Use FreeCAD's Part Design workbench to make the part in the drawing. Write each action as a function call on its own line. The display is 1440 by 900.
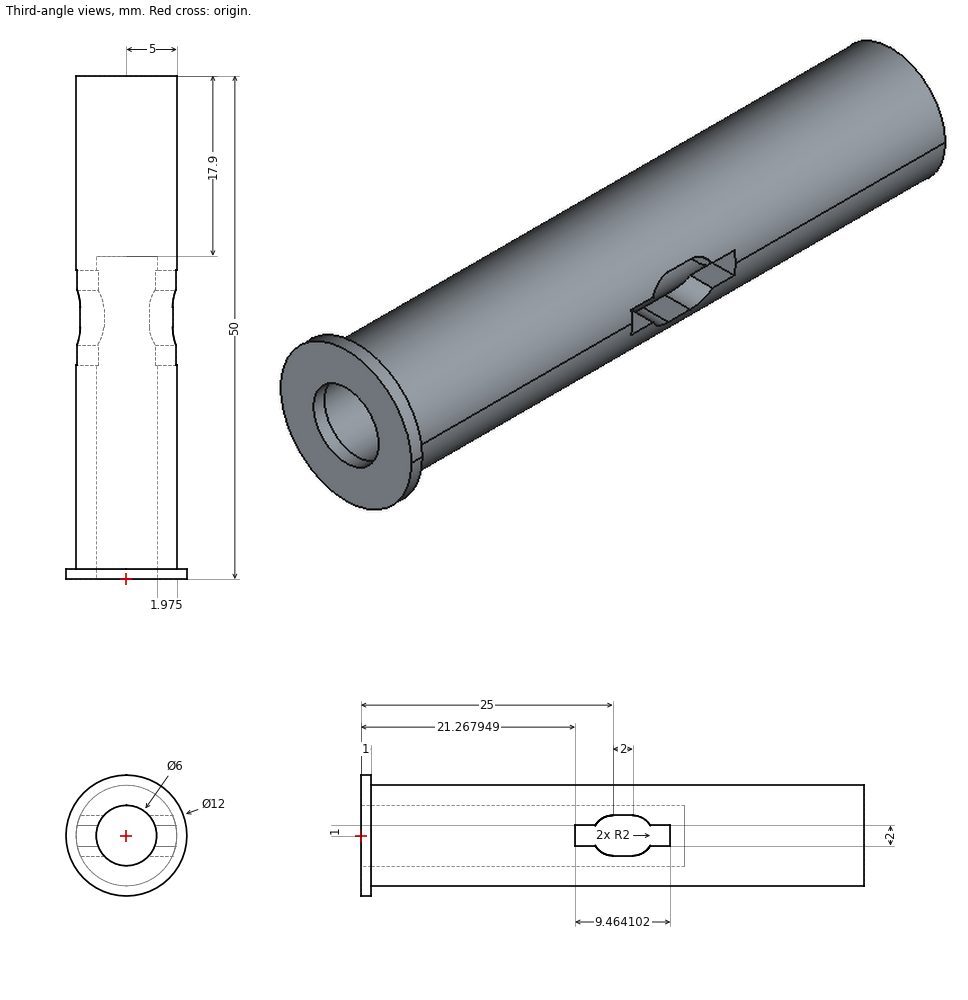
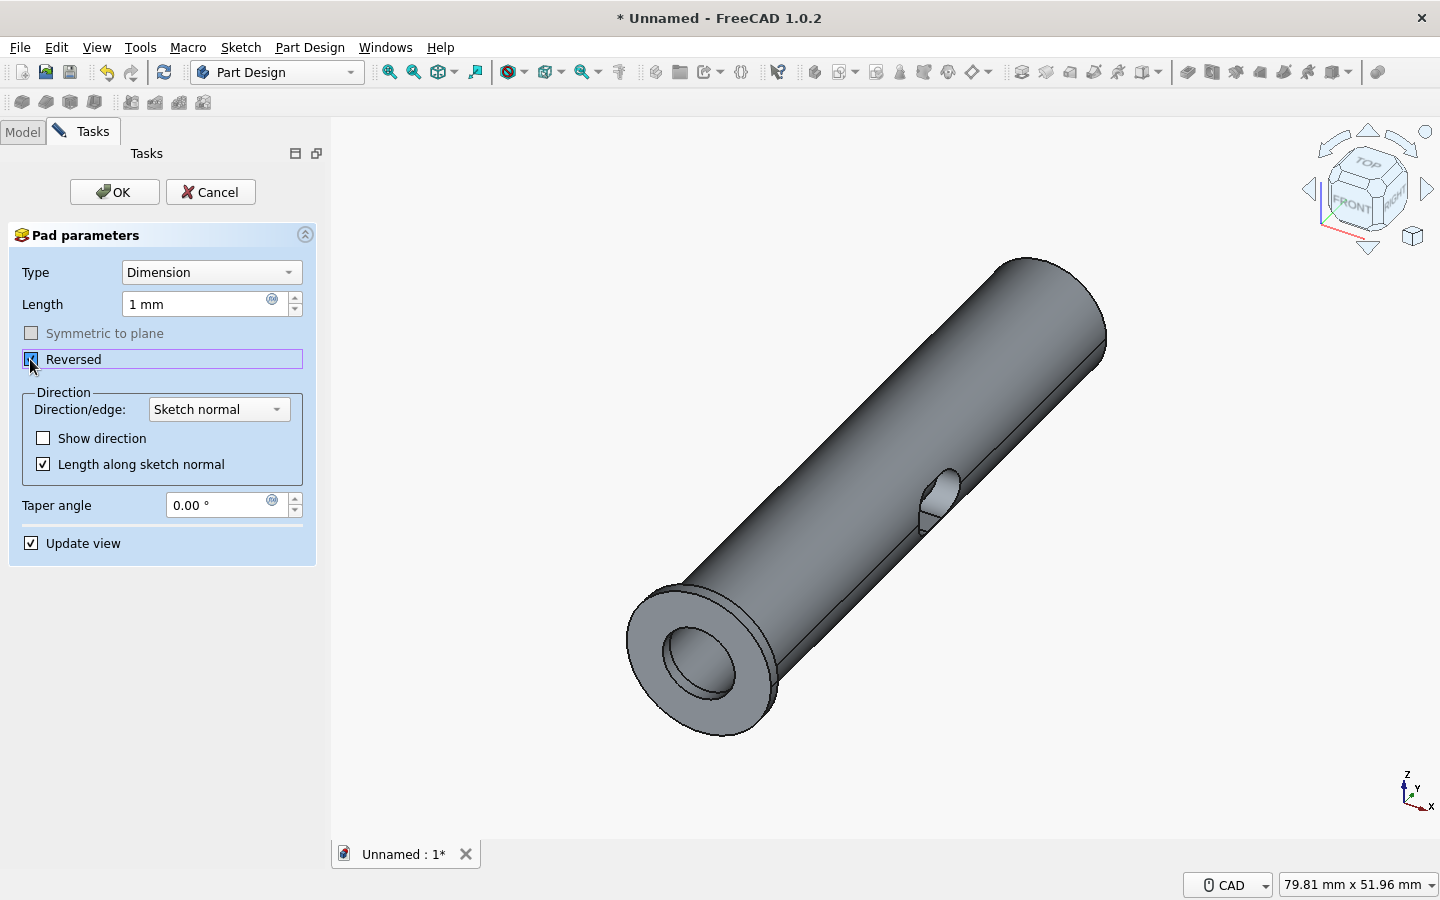
click(115, 192)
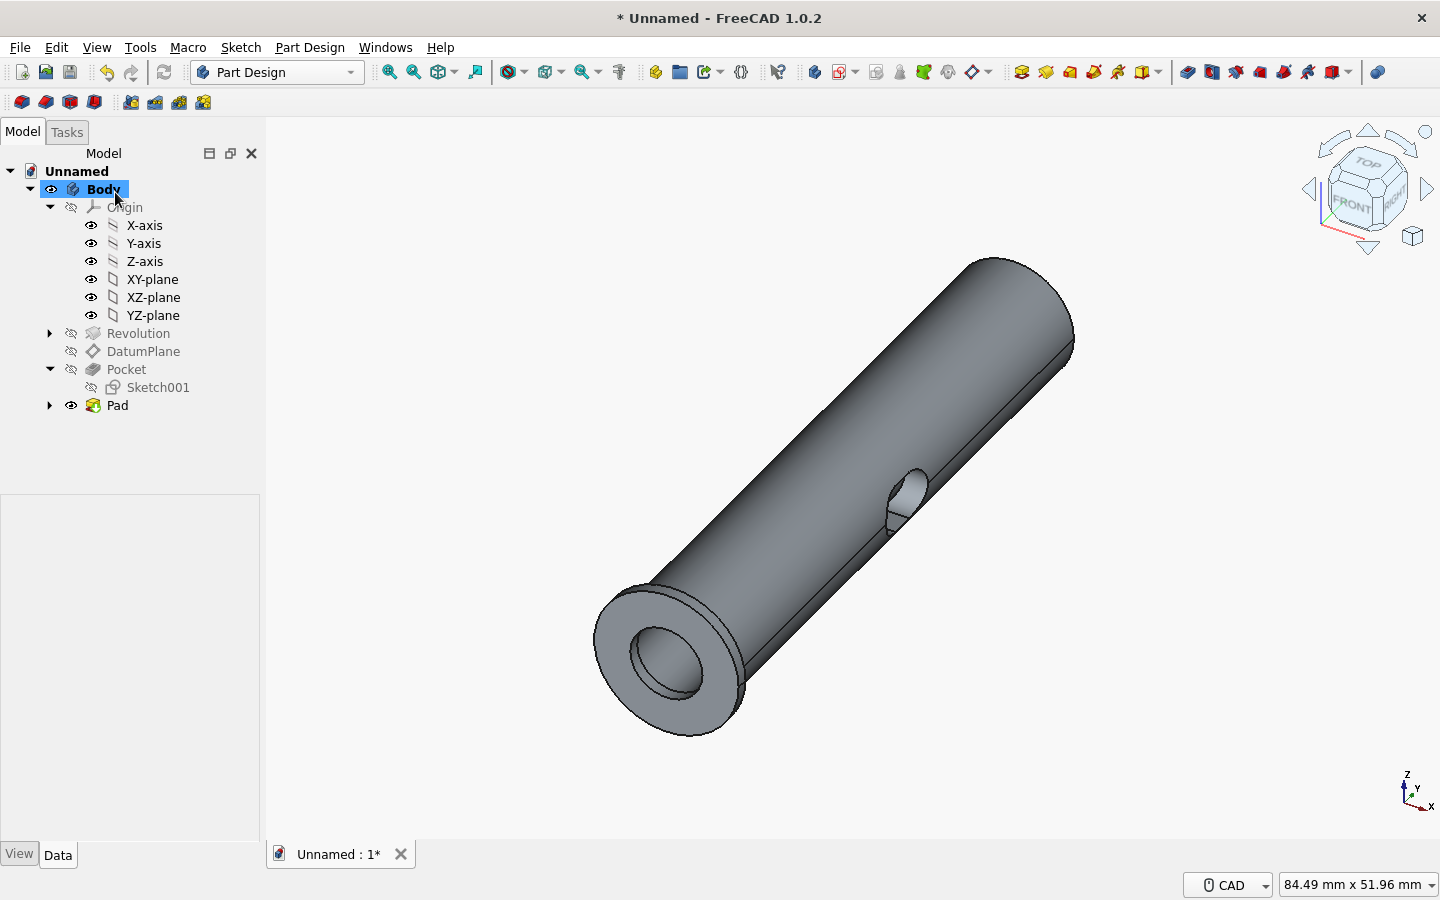
click(136, 315)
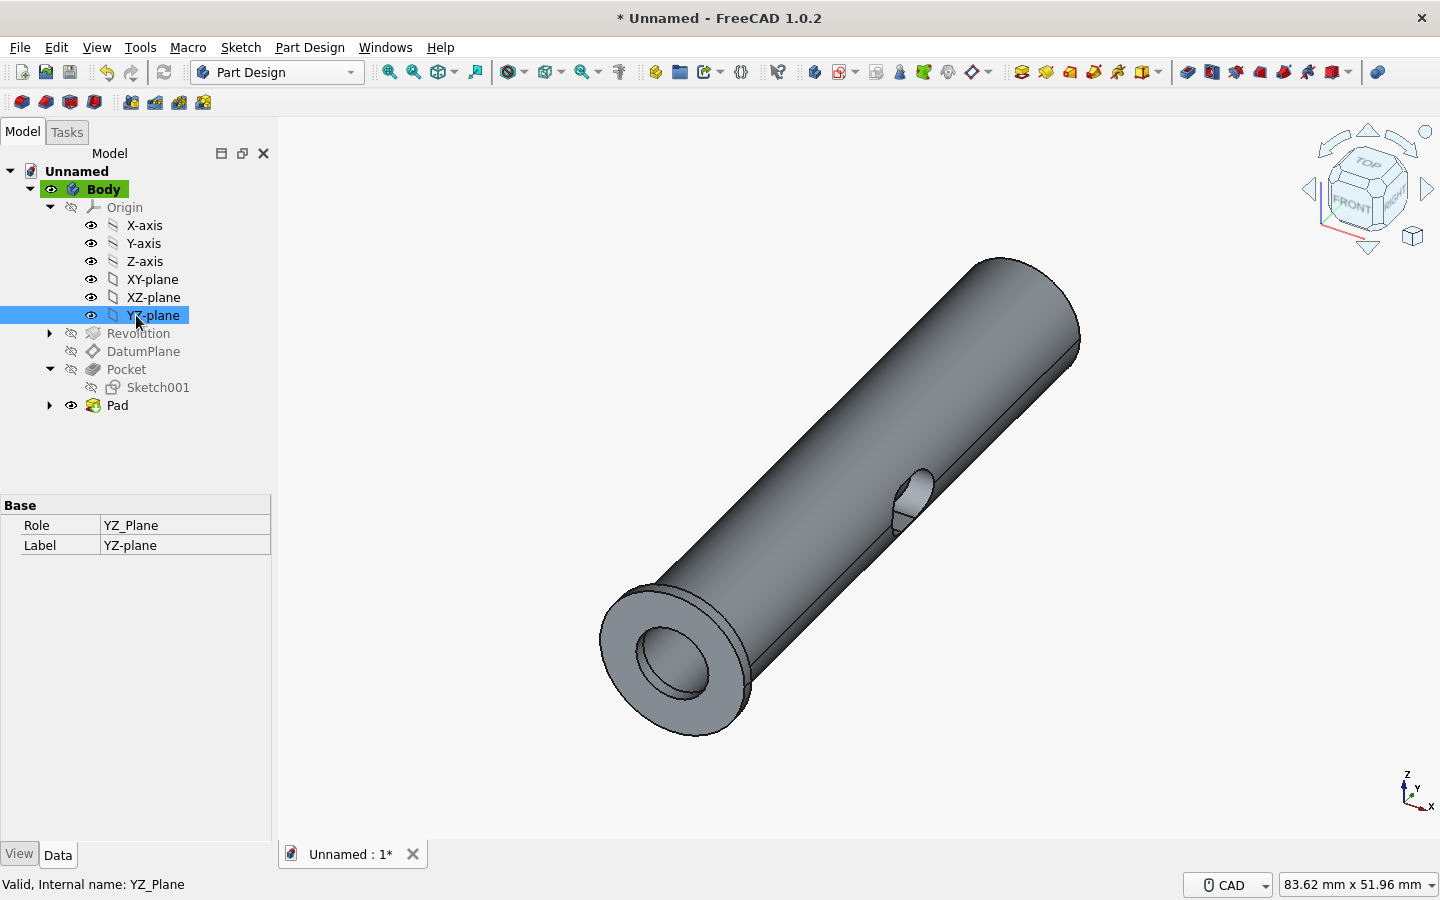
click(972, 72)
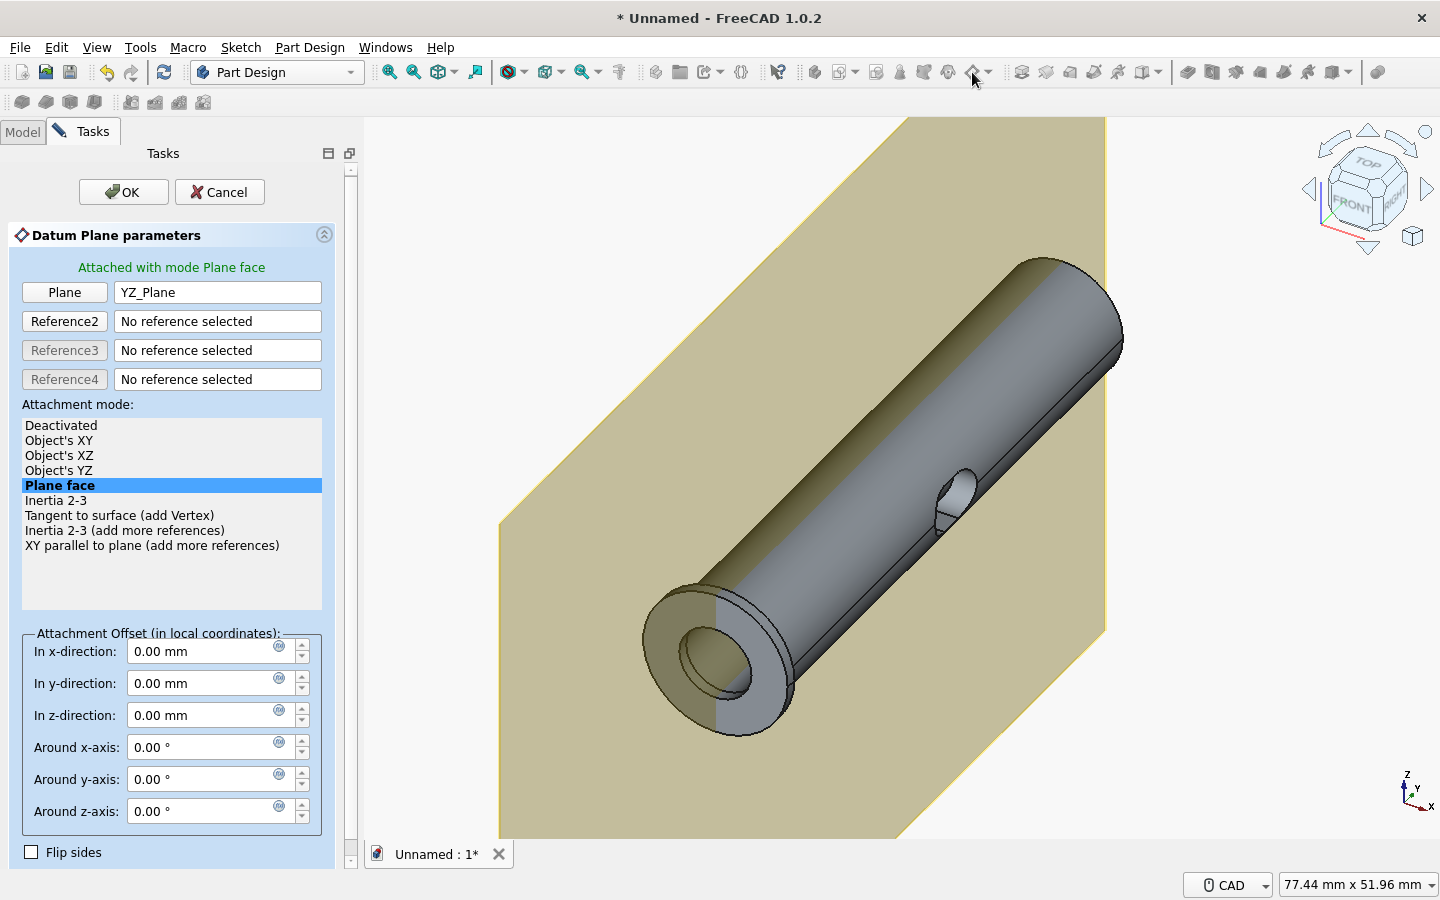
triple_click(210, 715)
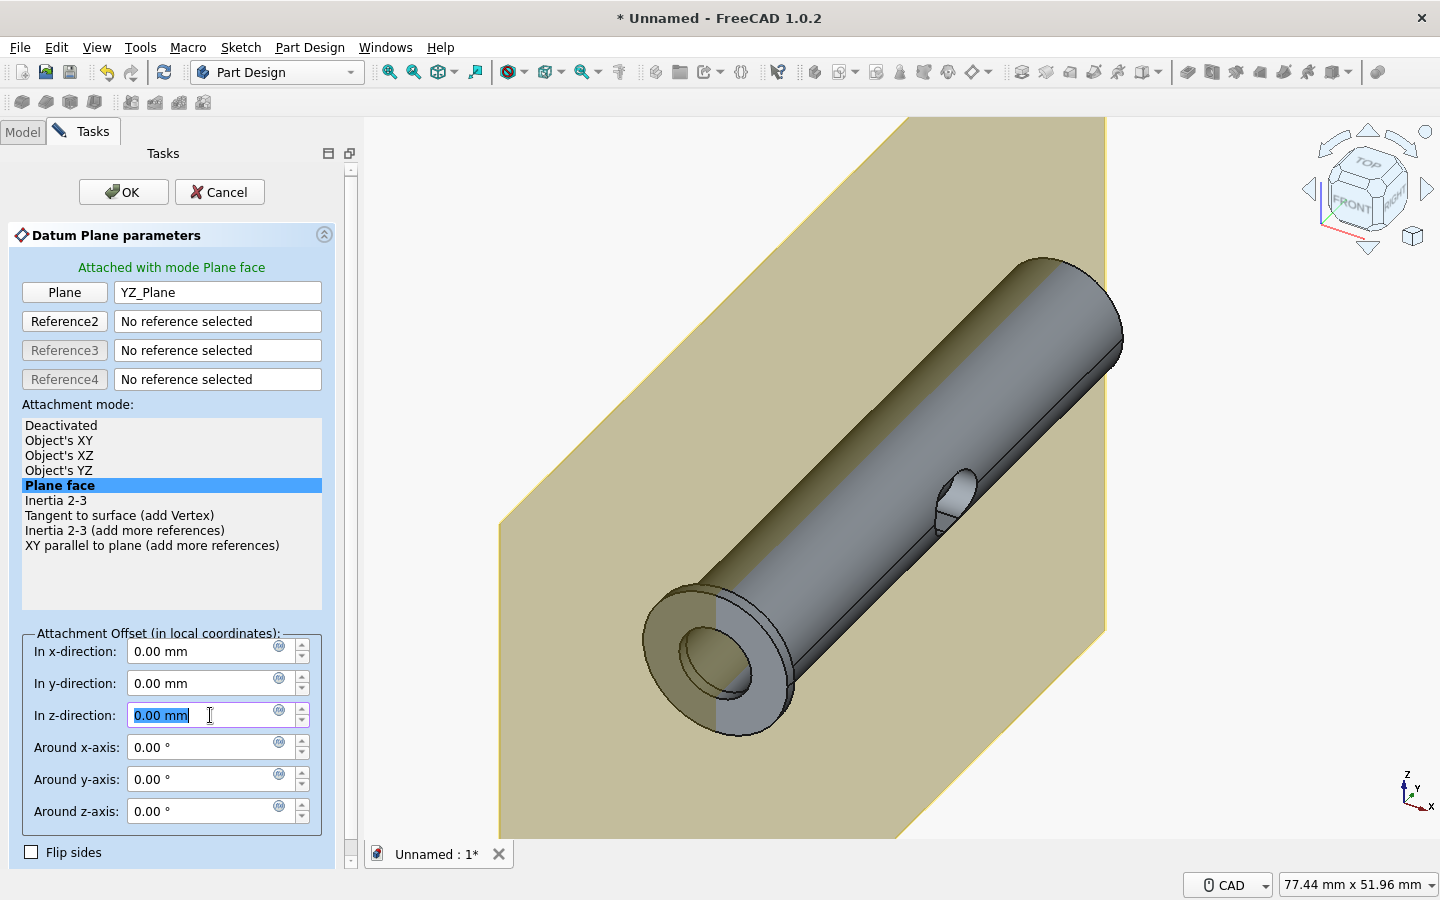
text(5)
key(Tab)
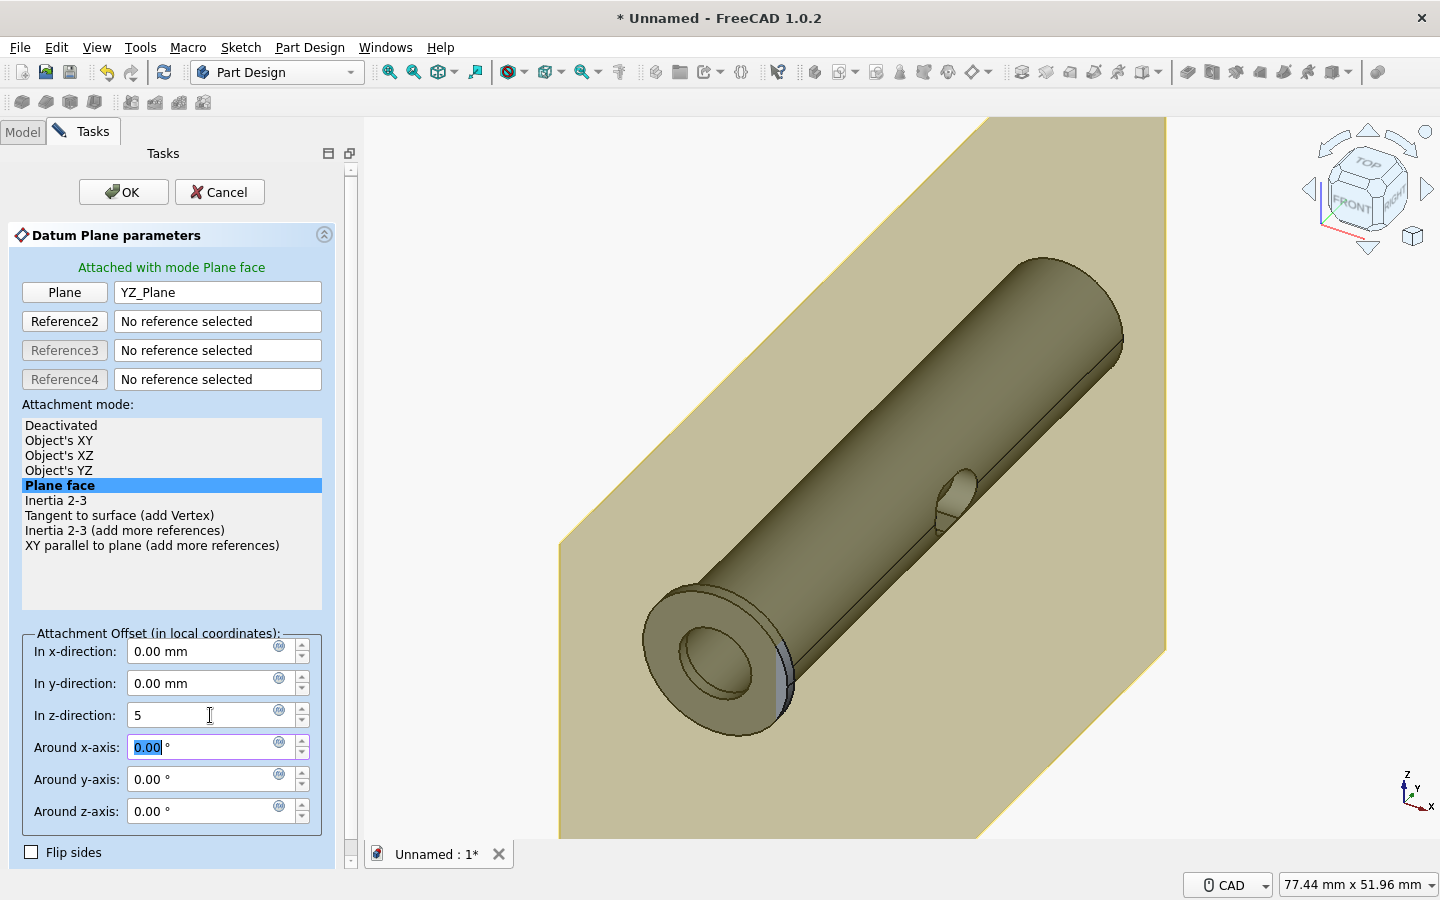
click(124, 192)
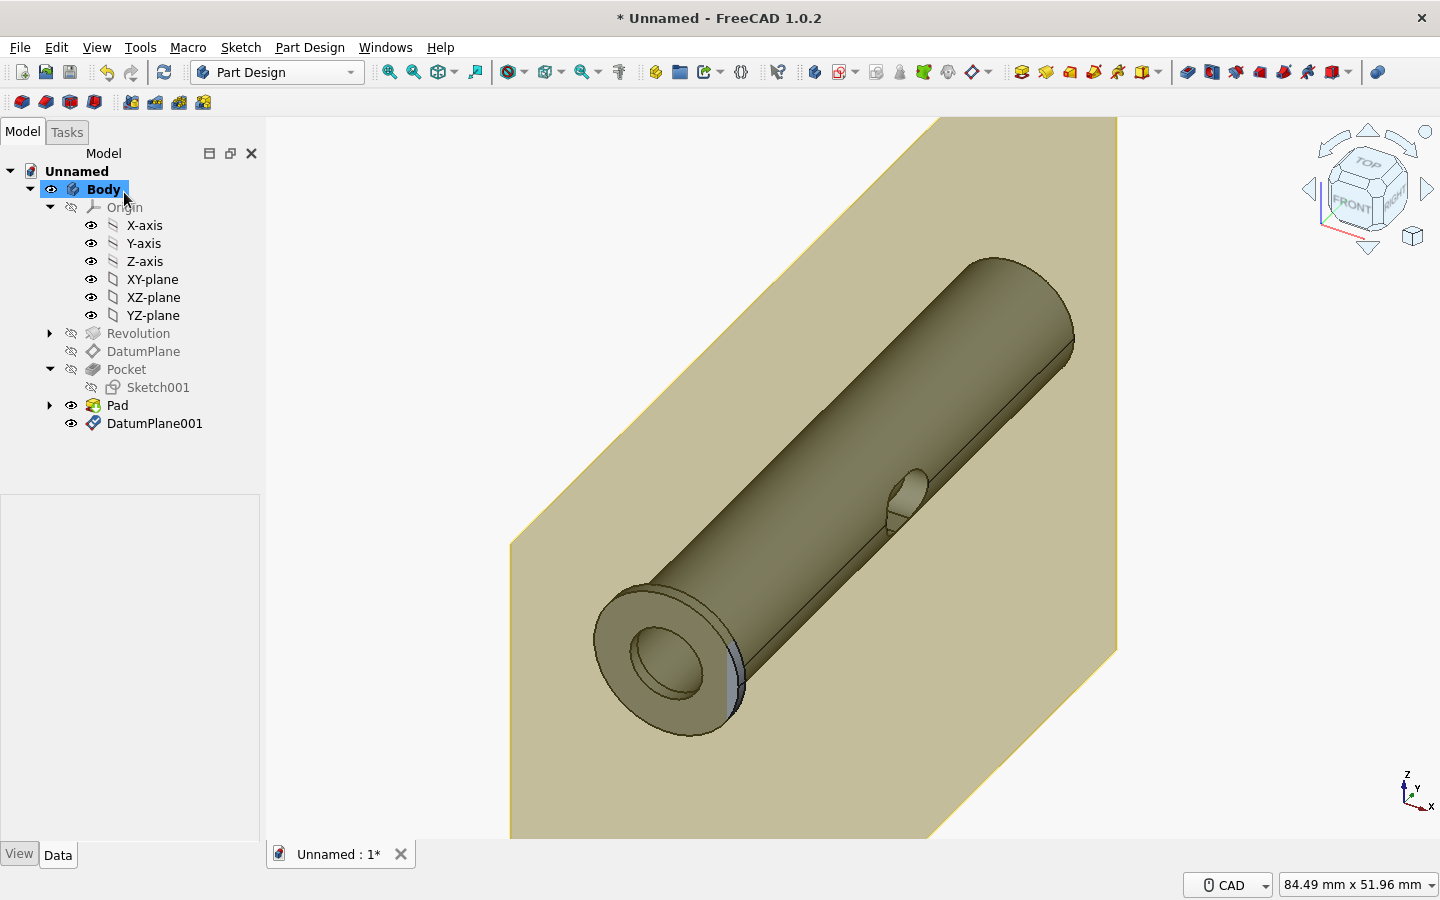
click(116, 423)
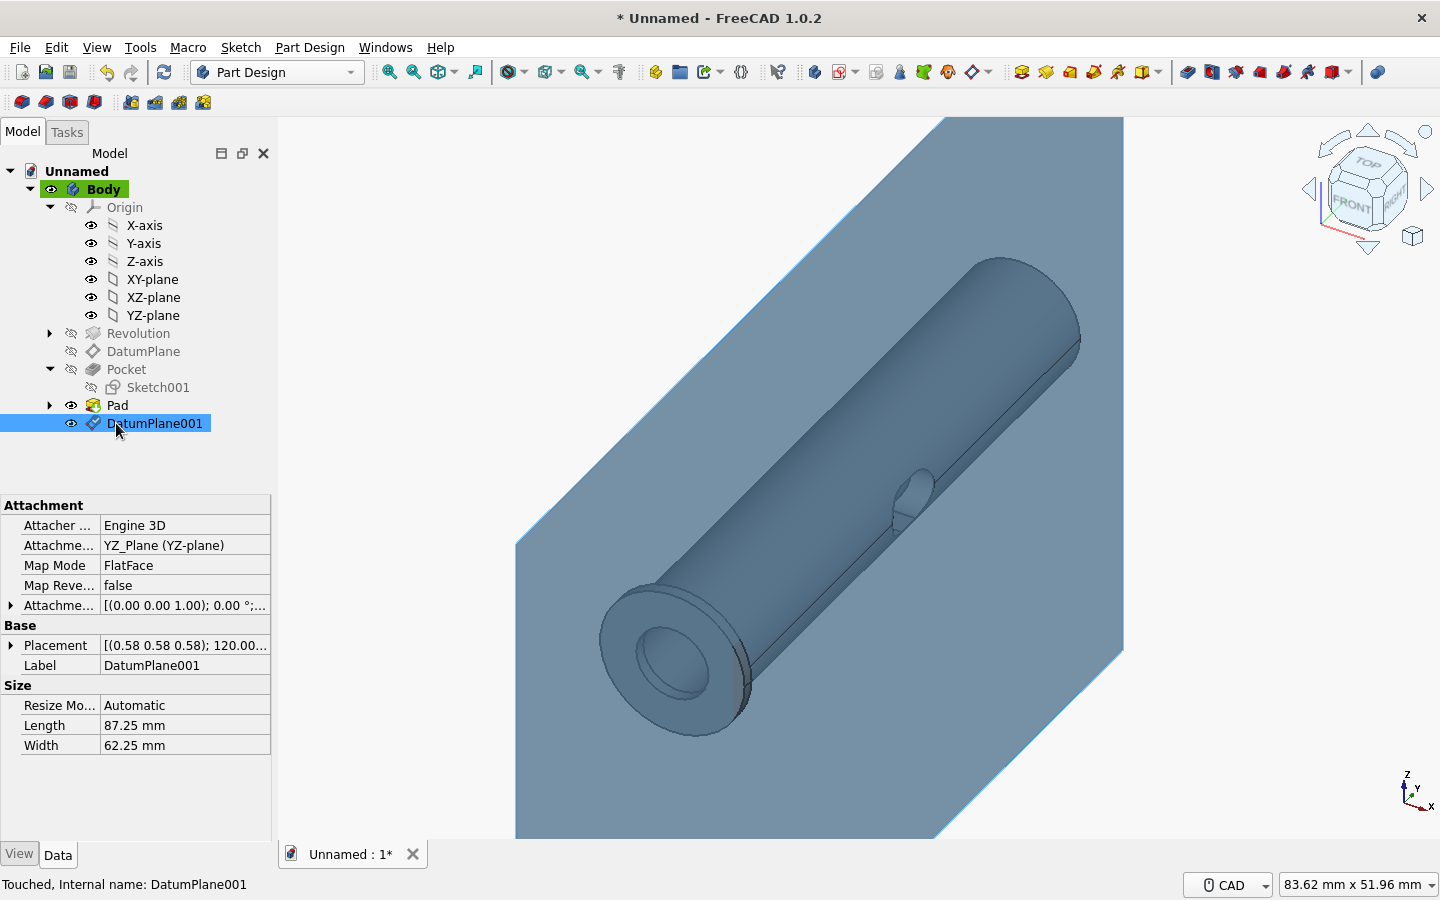
click(840, 72)